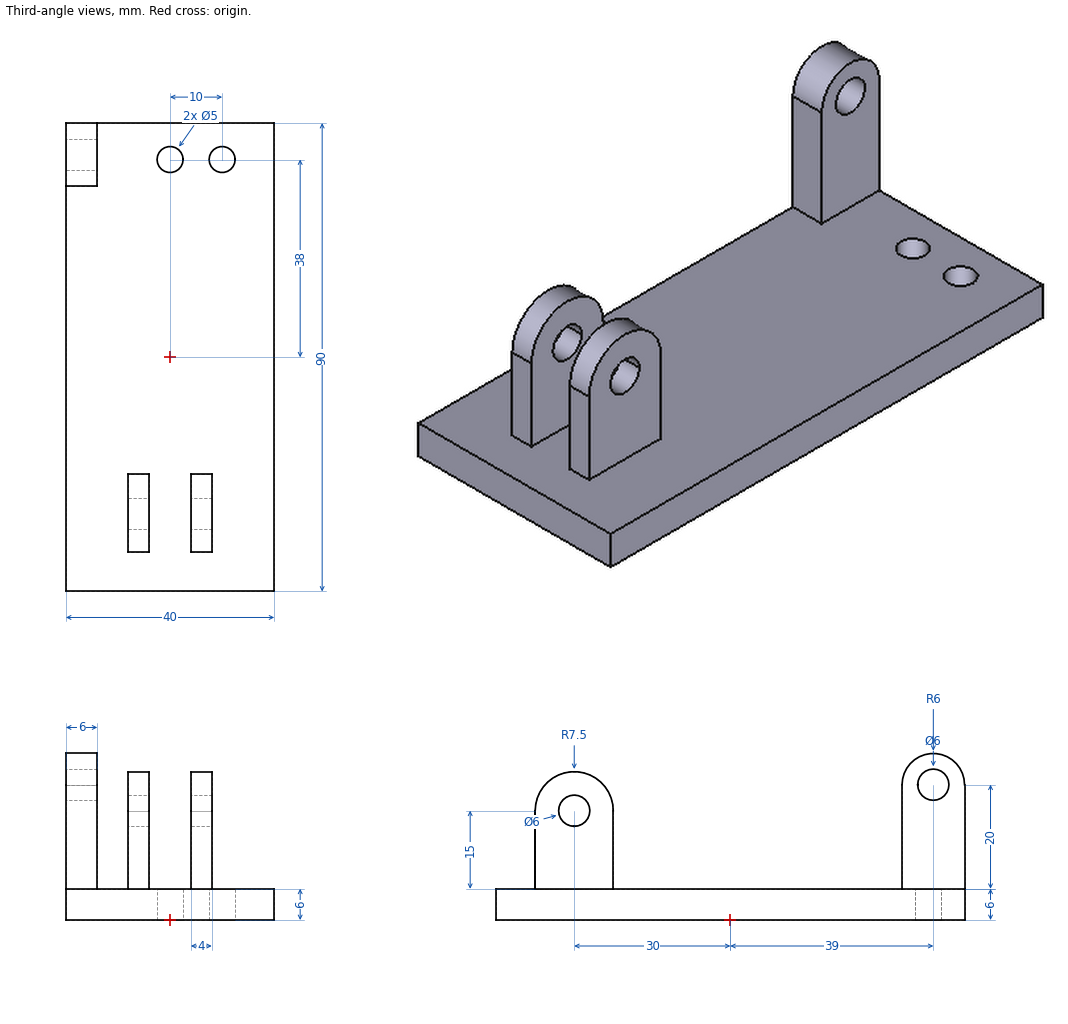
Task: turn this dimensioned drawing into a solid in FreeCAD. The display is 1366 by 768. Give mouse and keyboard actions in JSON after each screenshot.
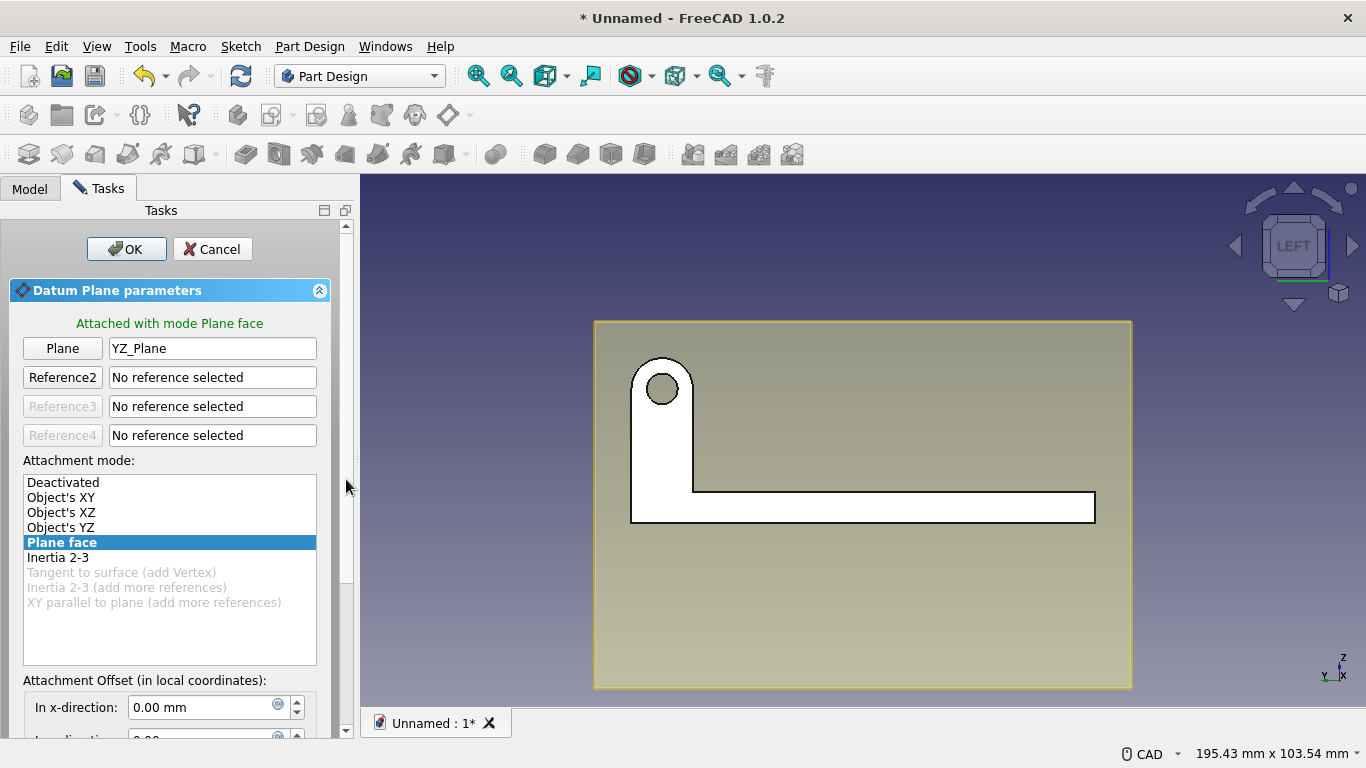
{"action": "left_click", "coordinate": [127, 249]}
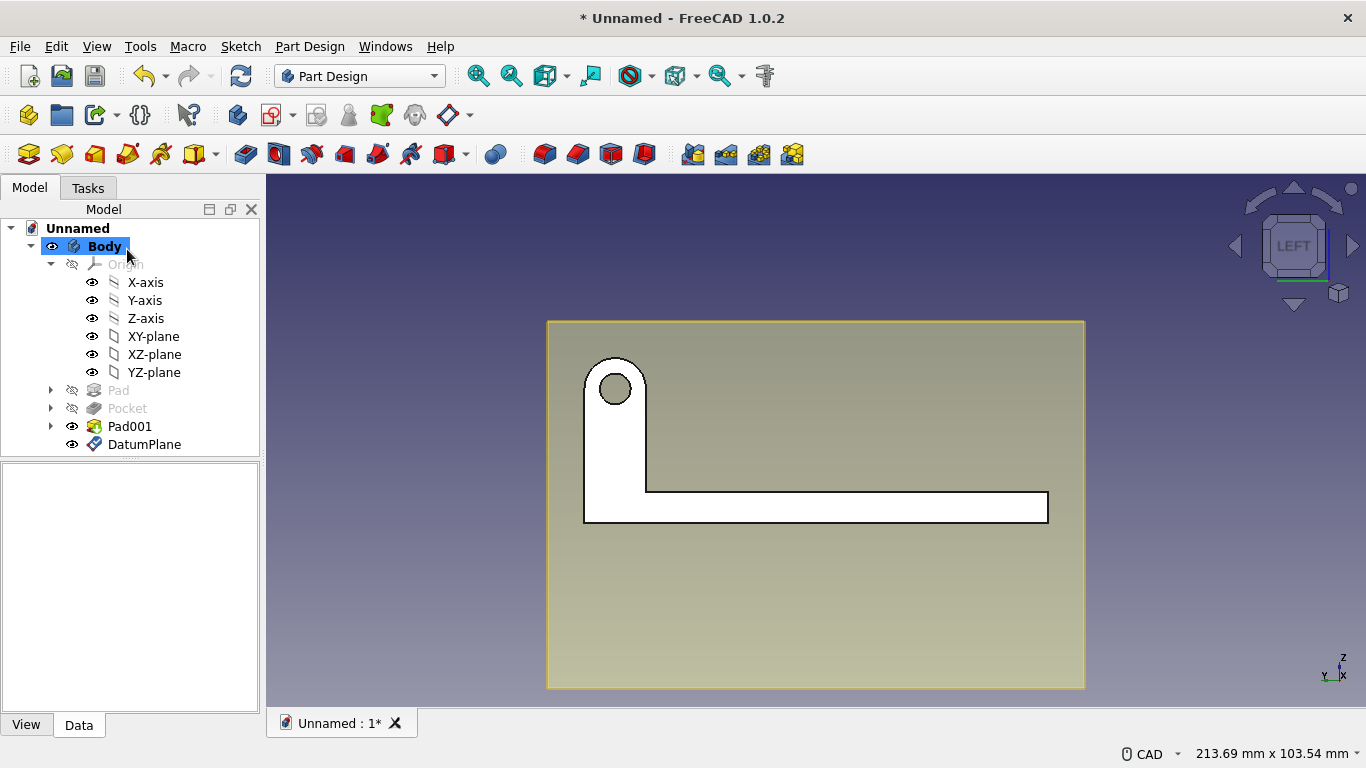
{"action": "left_click", "coordinate": [117, 444]}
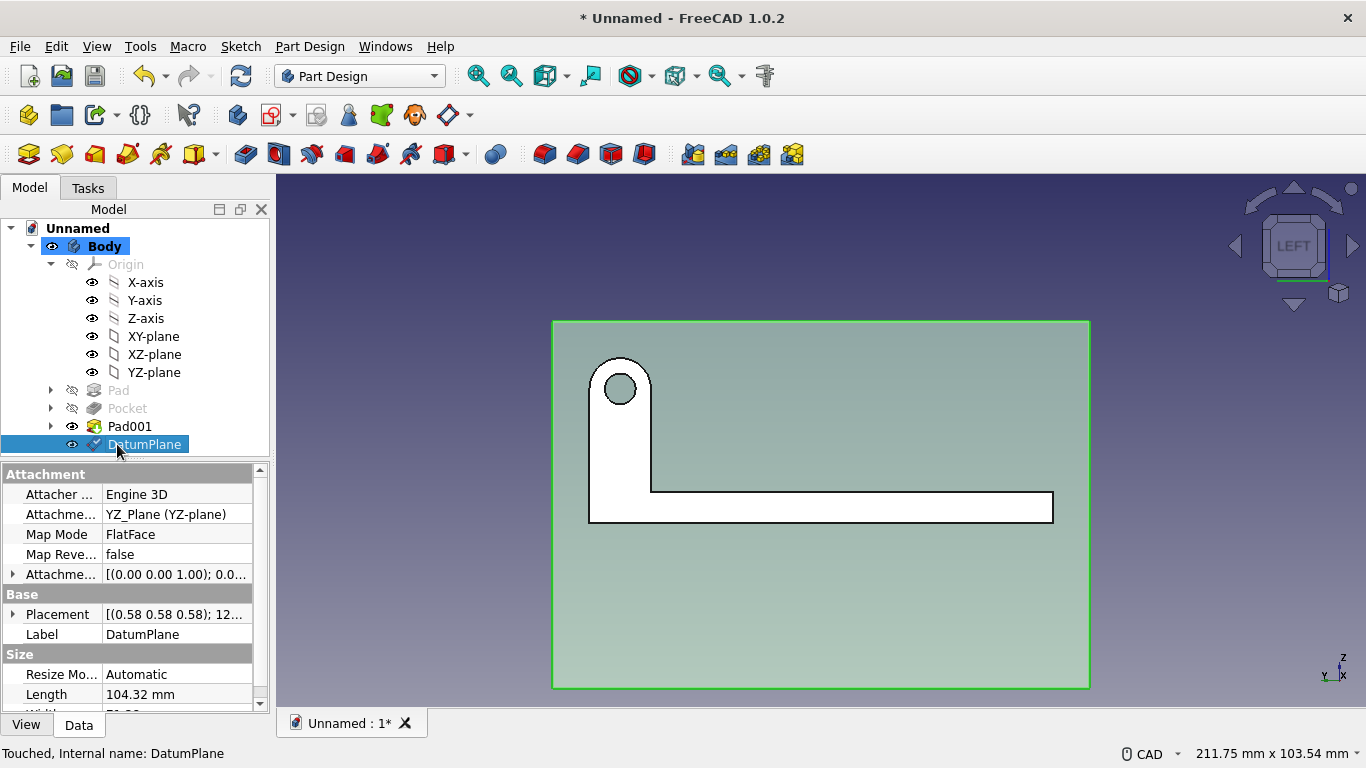
{"action": "left_click", "coordinate": [270, 116]}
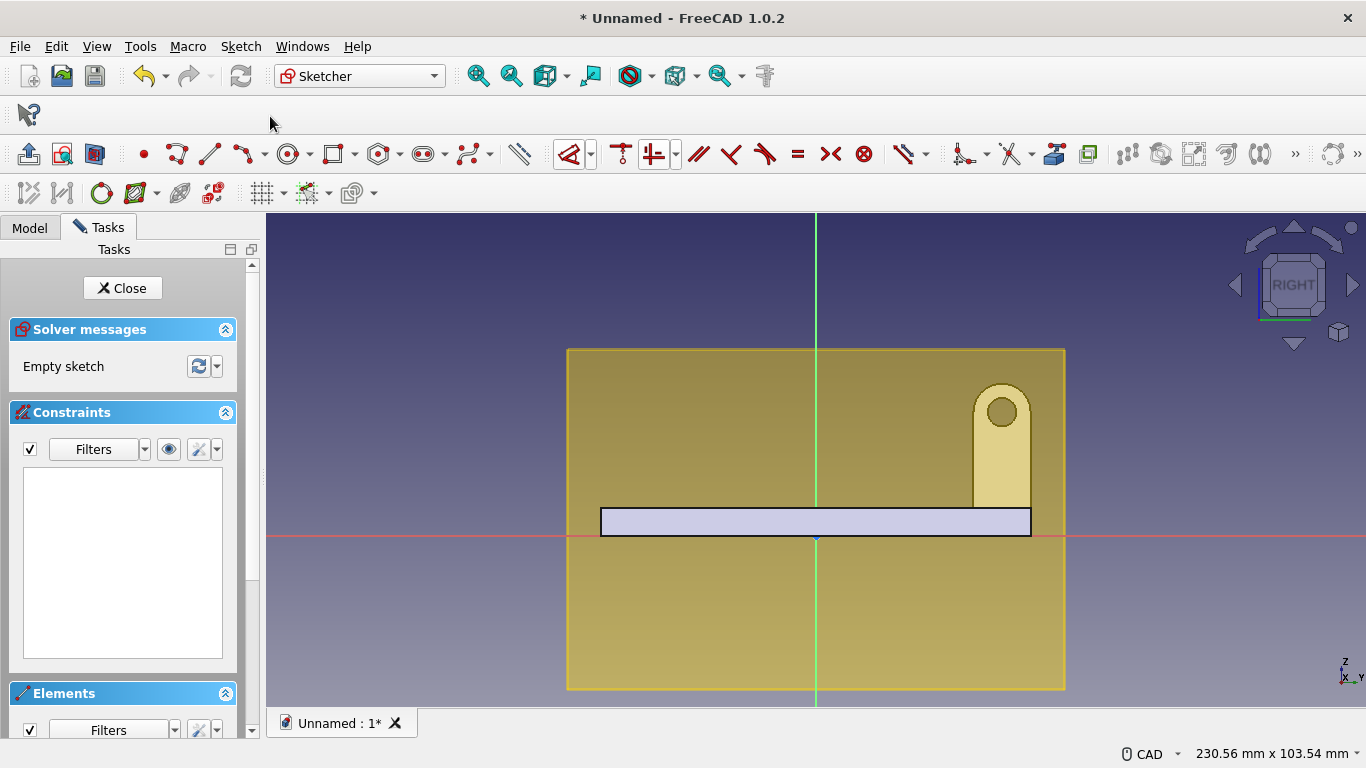
{"action": "key", "text": "q s"}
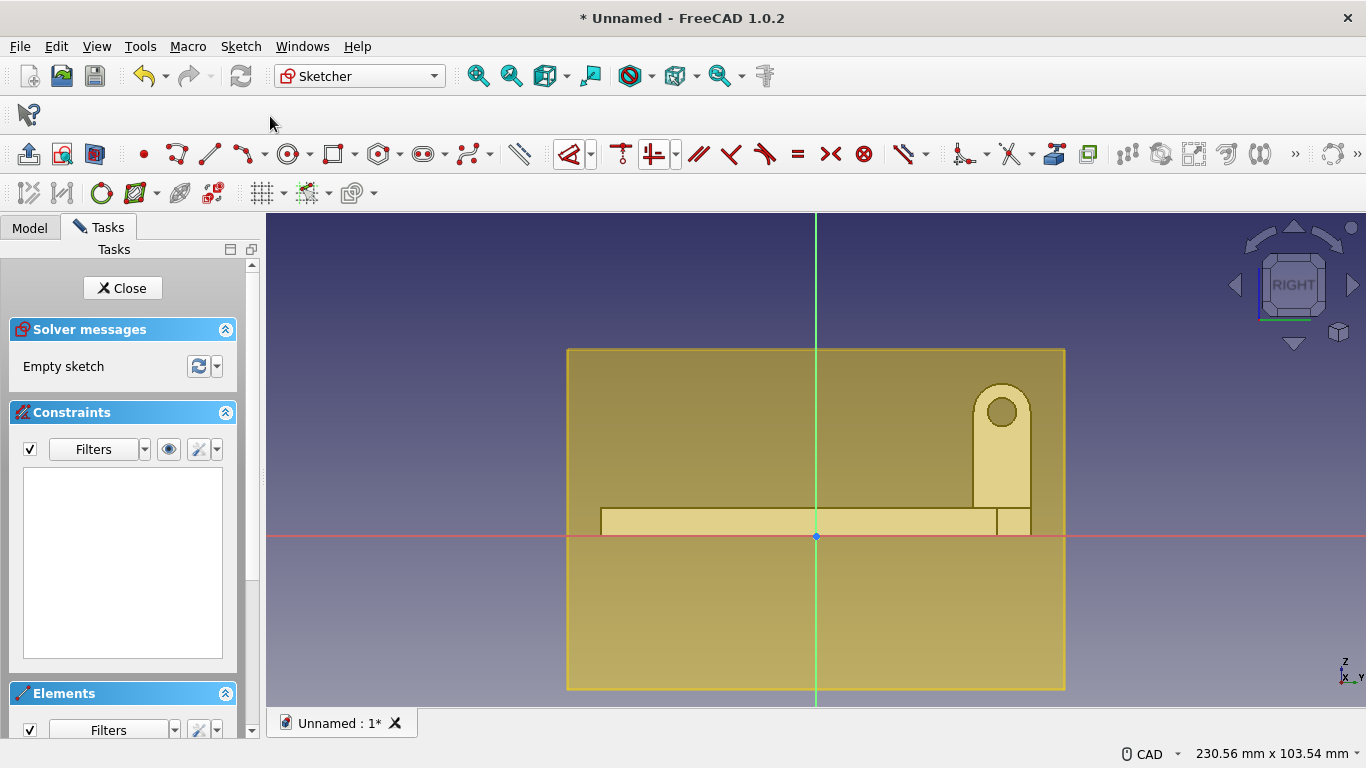
{"action": "scroll", "coordinate": [709, 475], "scroll_direction": "up", "scroll_amount": 4}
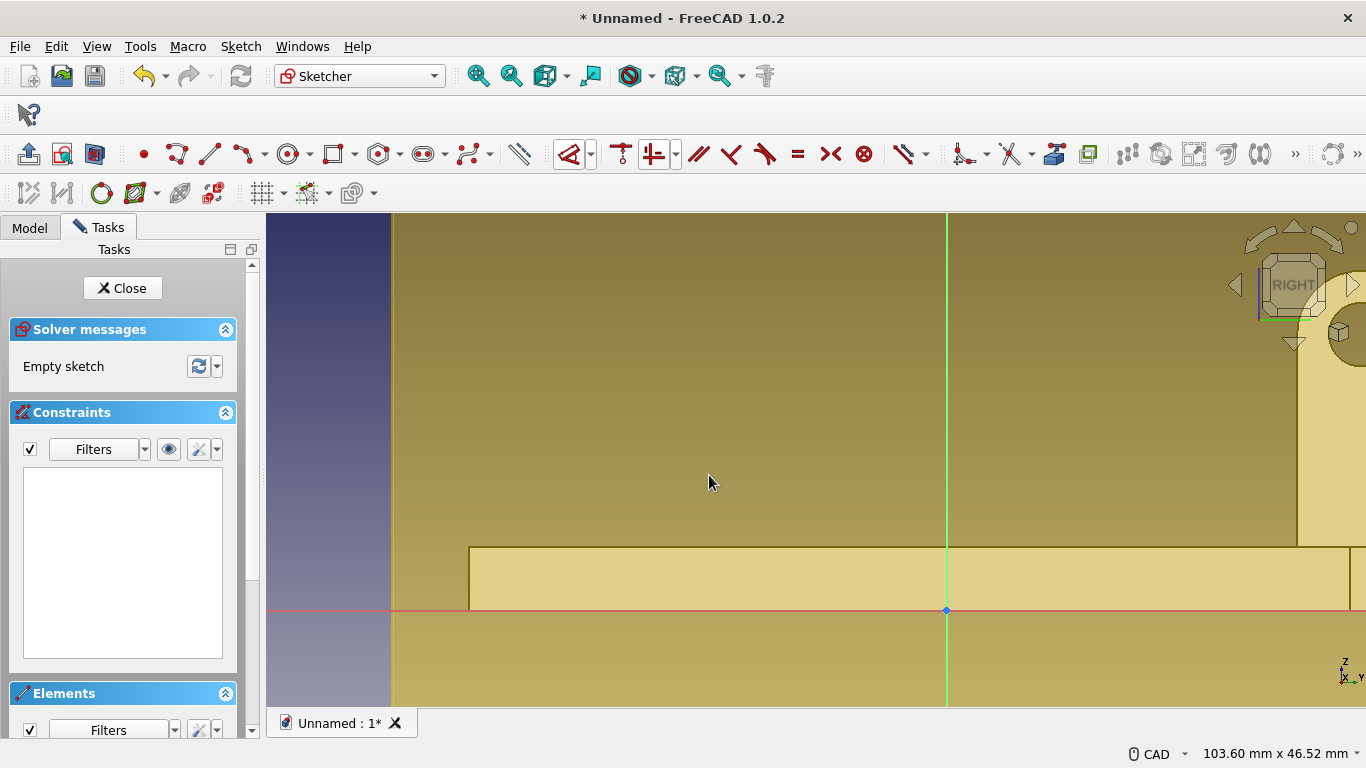
{"action": "key", "text": "g m"}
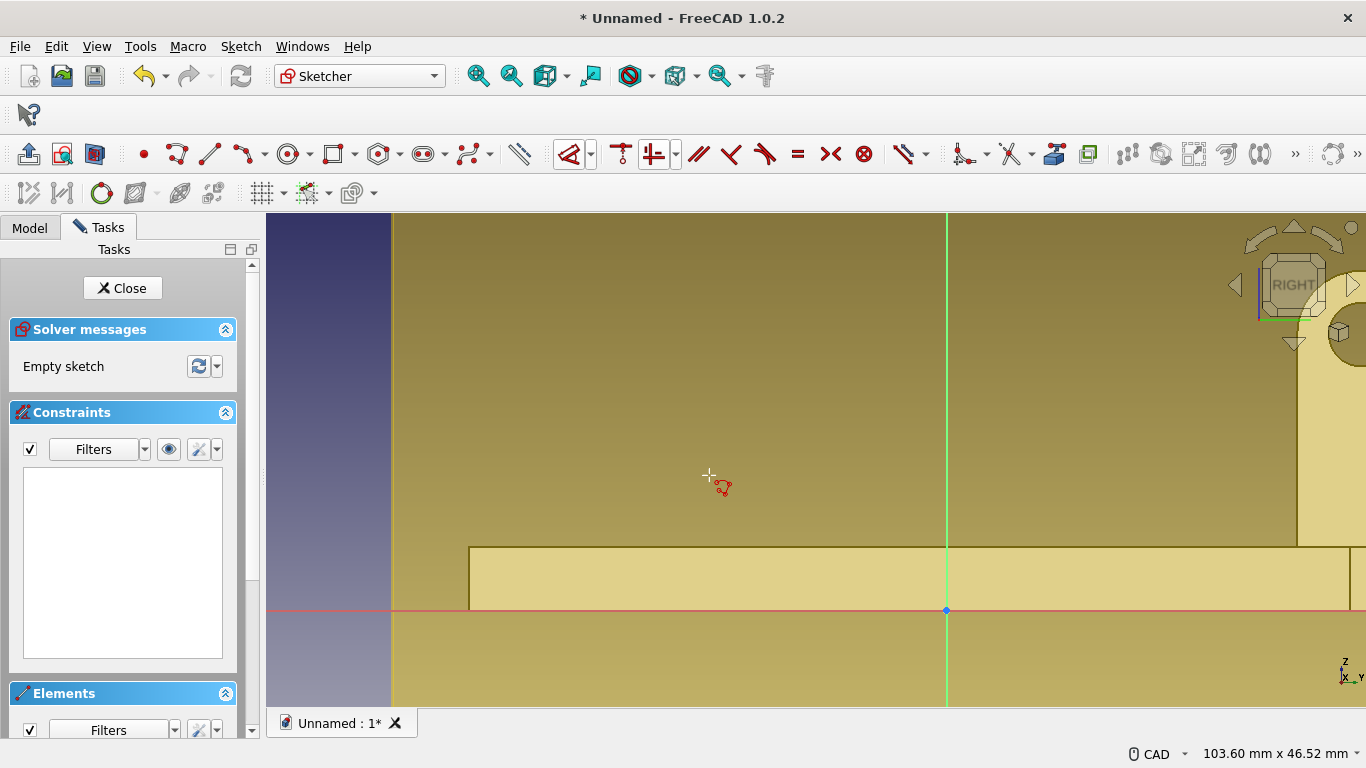
{"action": "left_click", "coordinate": [548, 388]}
{"action": "left_click", "coordinate": [548, 547]}
{"action": "left_click", "coordinate": [708, 547]}
{"action": "left_click", "coordinate": [708, 388]}
{"action": "right_click", "coordinate": [708, 388]}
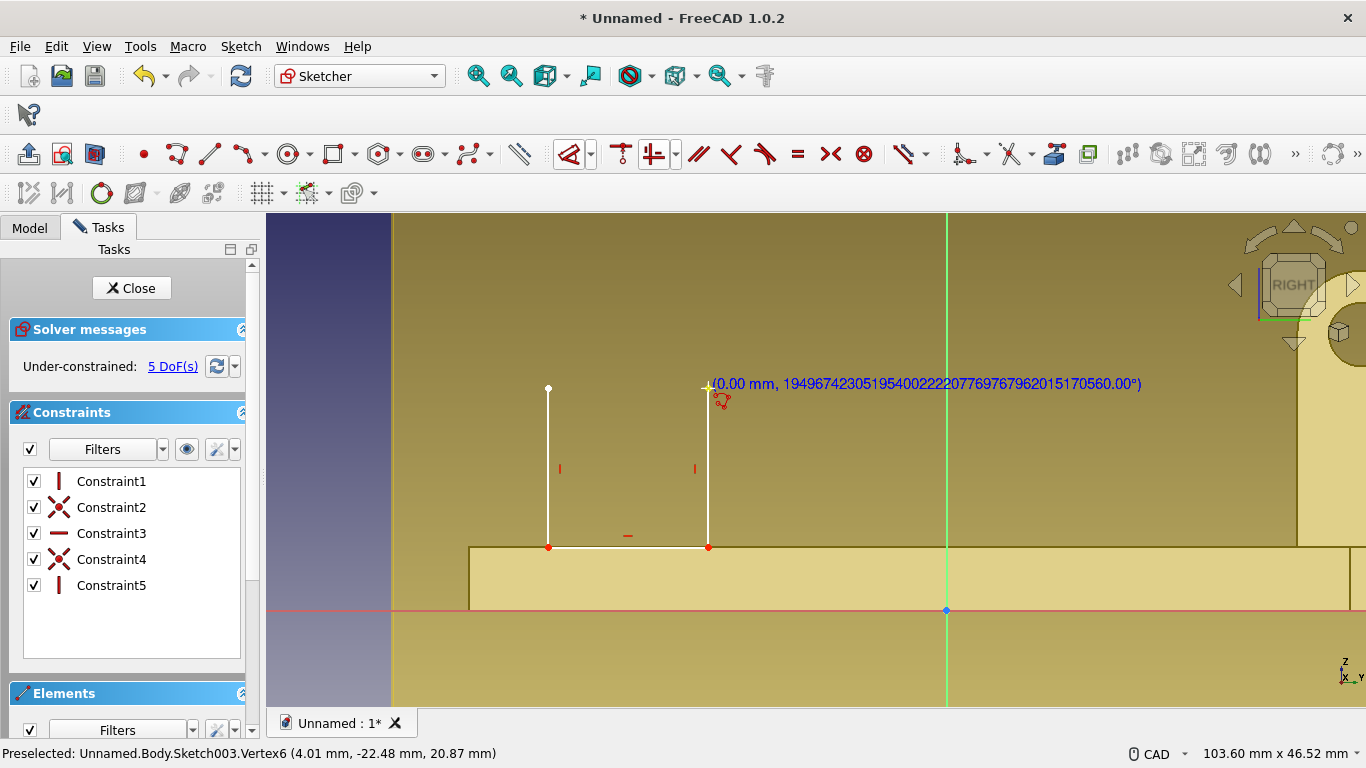
{"action": "key", "text": "g 3 a"}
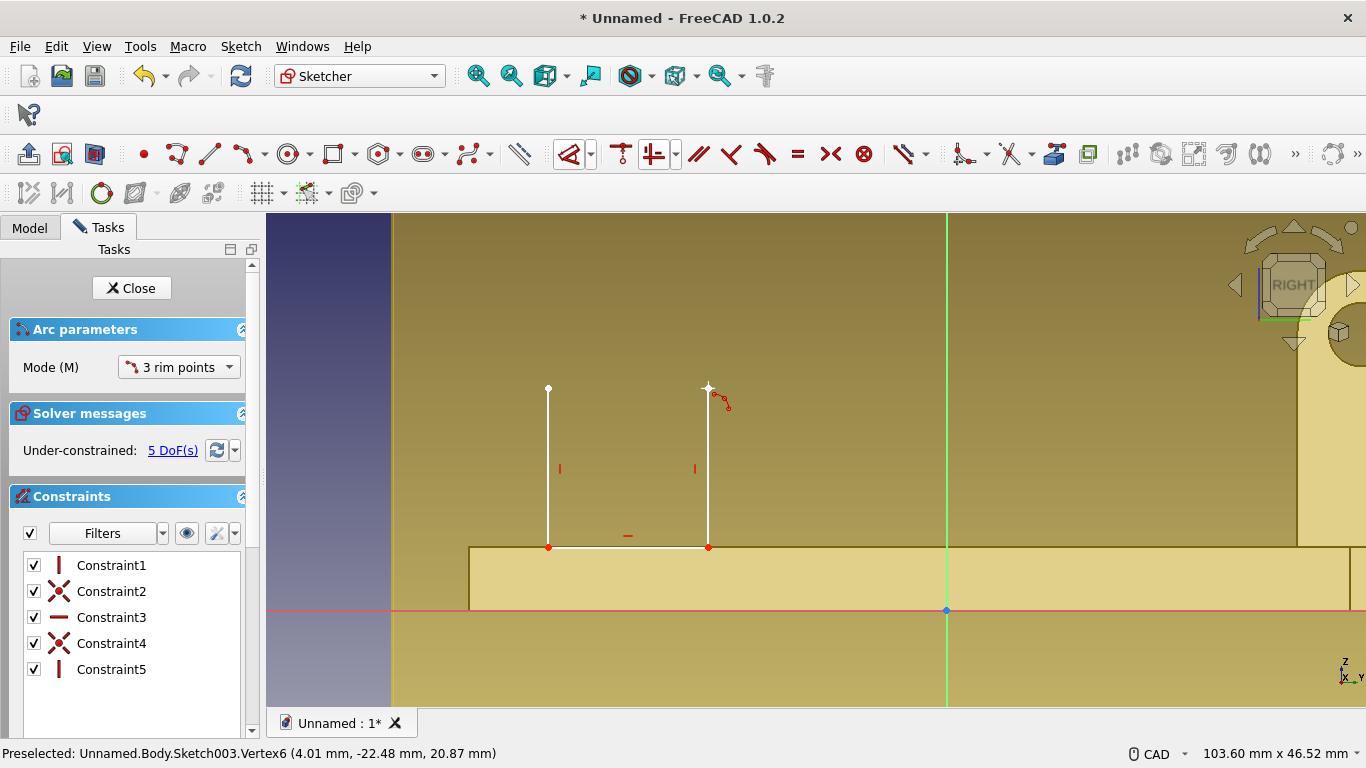
{"action": "left_click", "coordinate": [708, 389]}
{"action": "left_click", "coordinate": [548, 389]}
{"action": "left_click", "coordinate": [628, 308]}